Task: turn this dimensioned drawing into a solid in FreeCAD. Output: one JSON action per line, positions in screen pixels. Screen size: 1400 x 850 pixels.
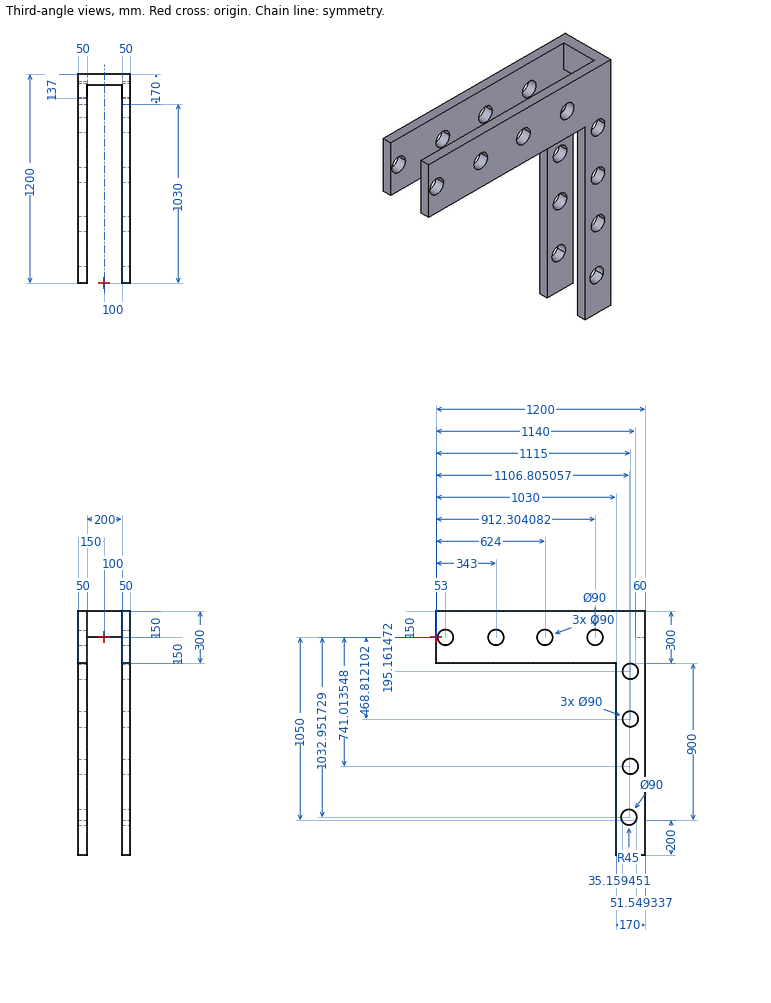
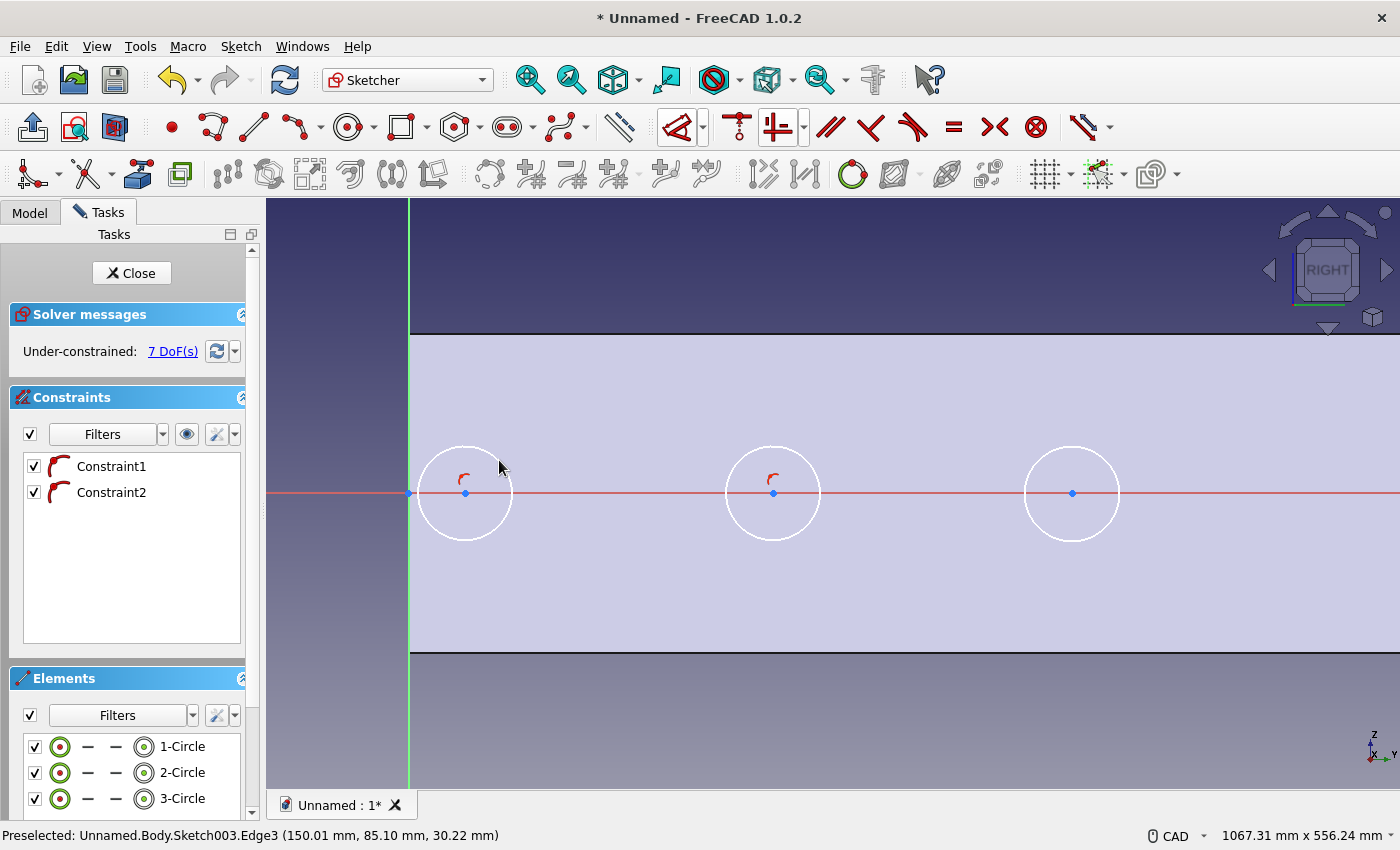
{"action": "left_click", "coordinate": [1105, 460]}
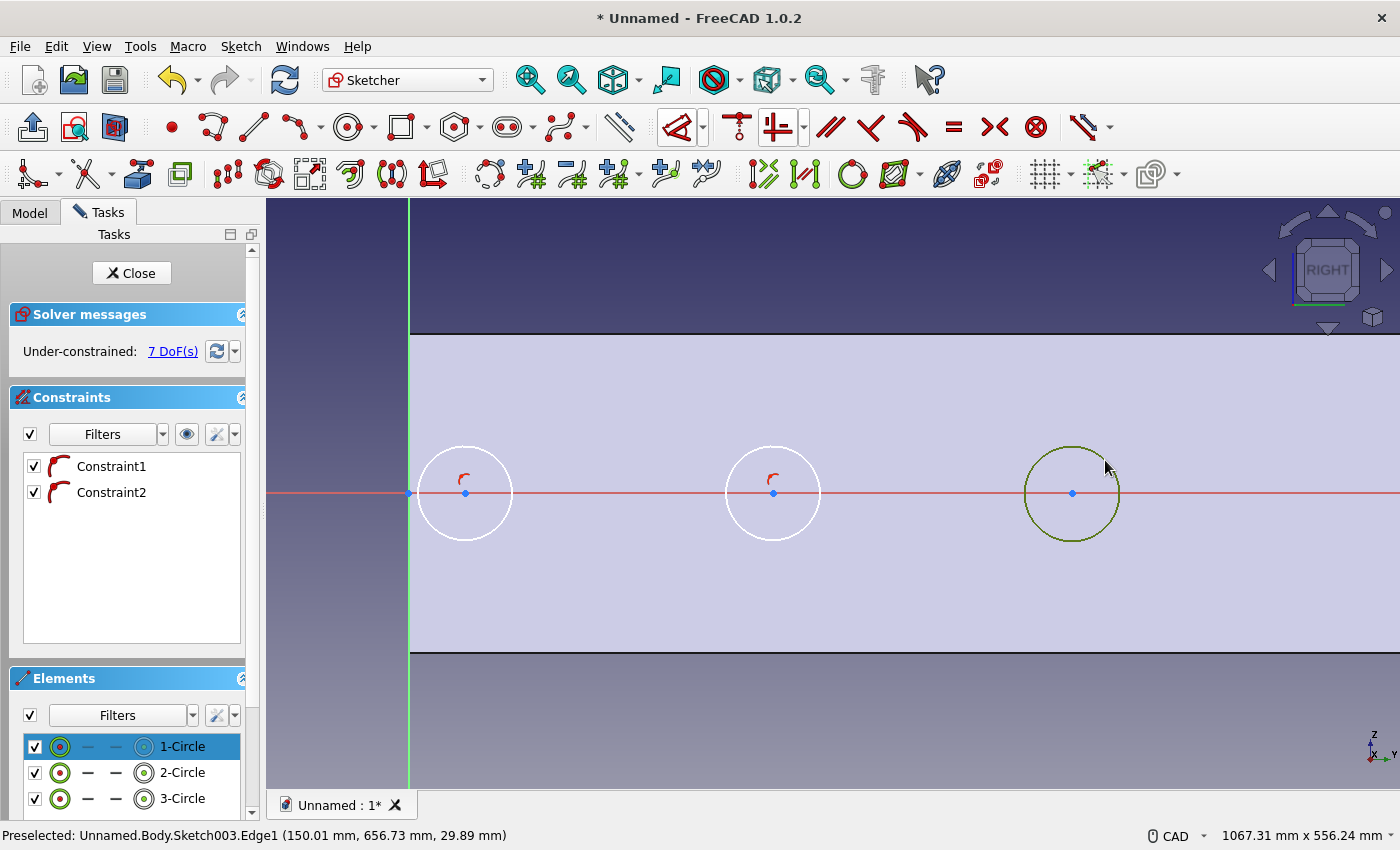
{"action": "left_click", "coordinate": [806, 460]}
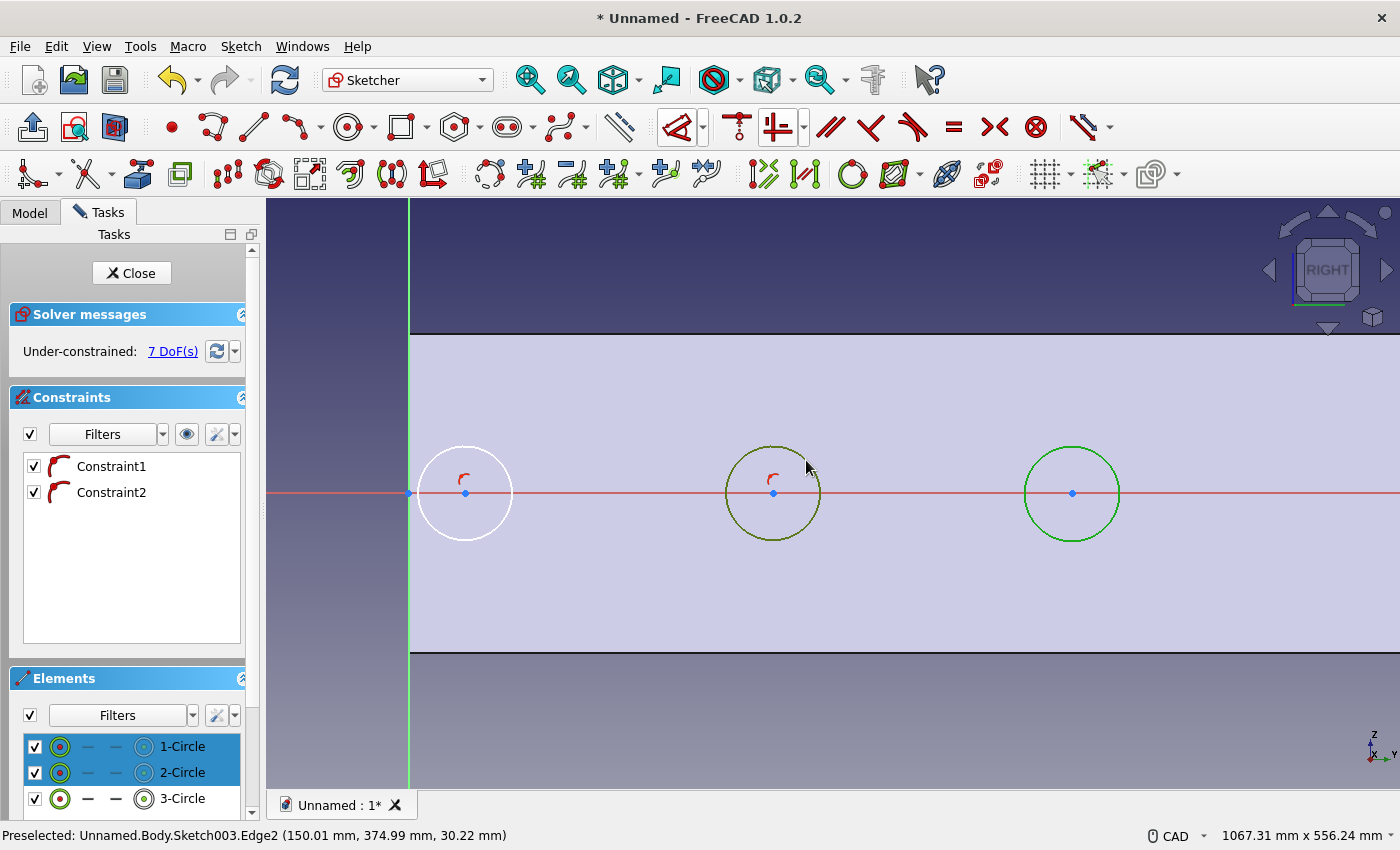
{"action": "left_click", "coordinate": [498, 460]}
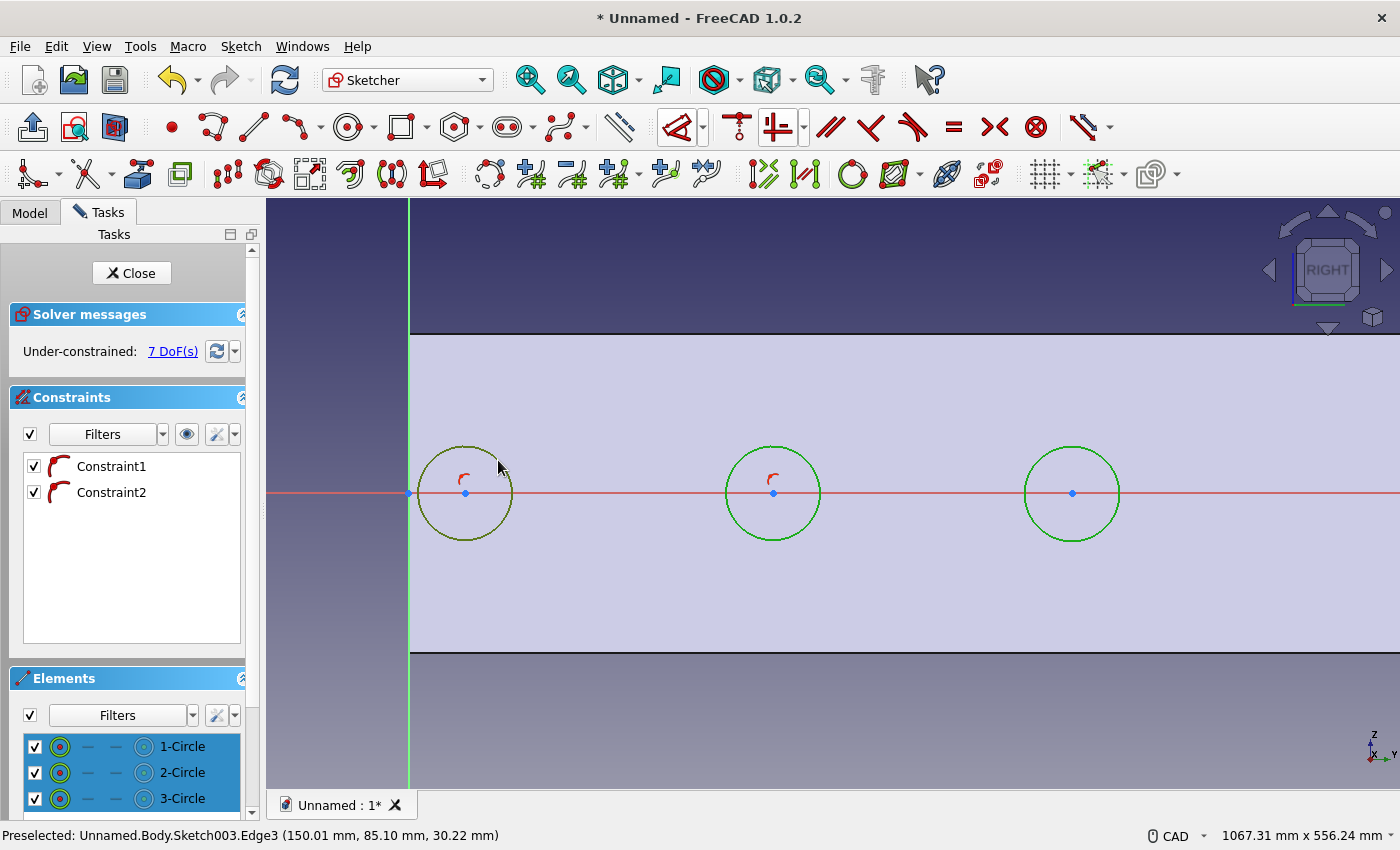
{"action": "left_click", "coordinate": [954, 128]}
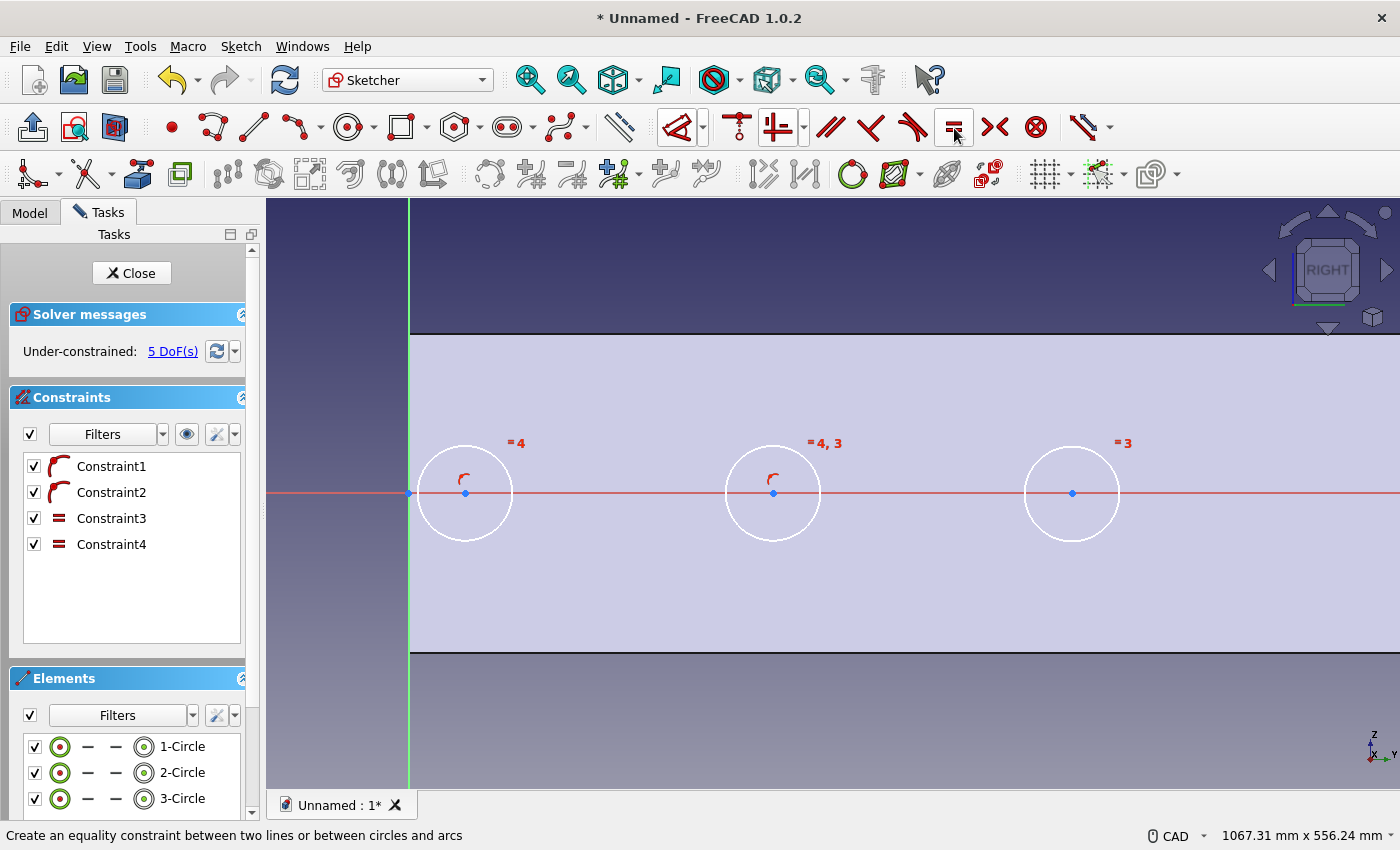
{"action": "left_click", "coordinate": [1072, 494]}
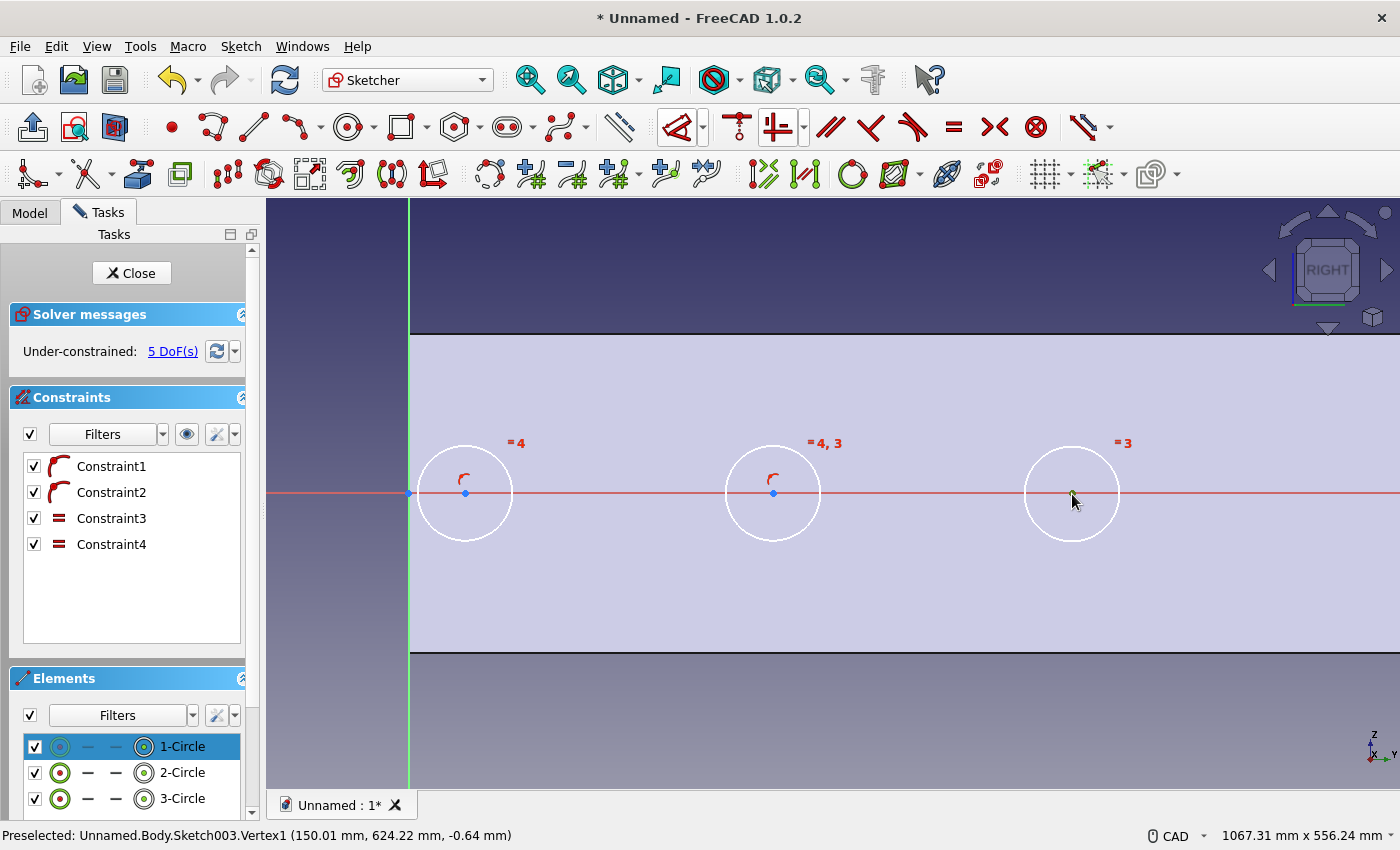
{"action": "left_click", "coordinate": [361, 493]}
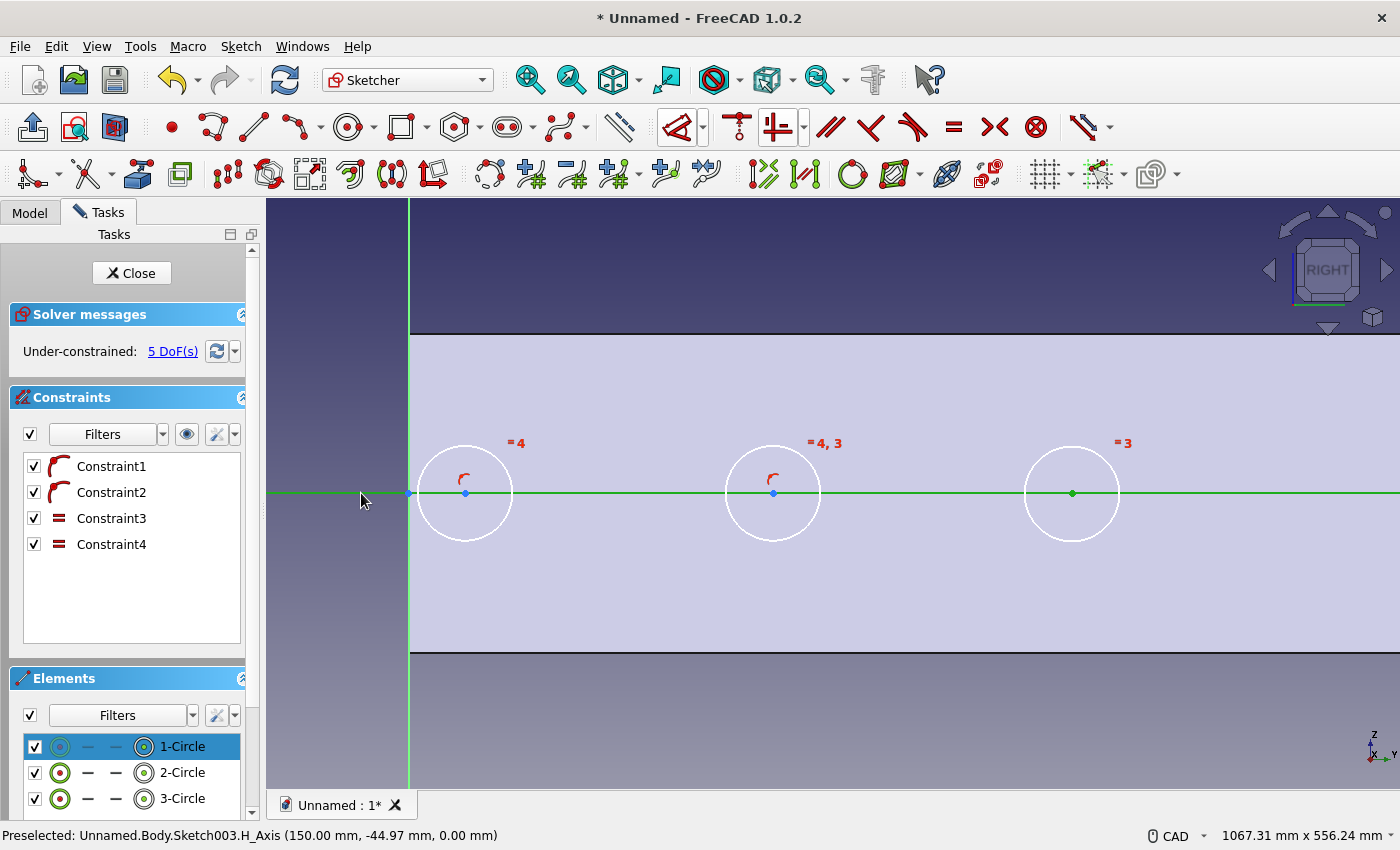
{"action": "left_click", "coordinate": [737, 128]}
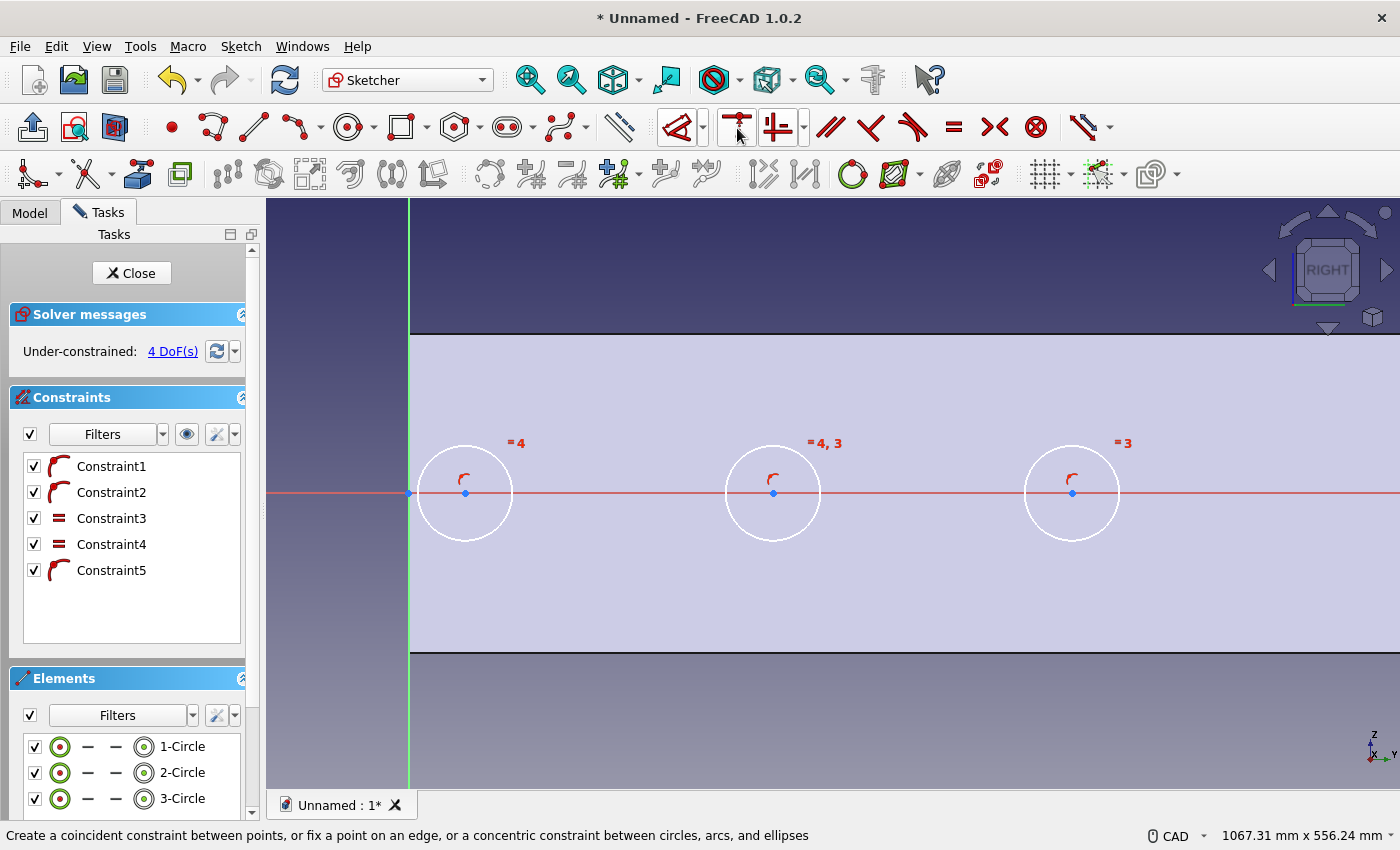
{"action": "left_click", "coordinate": [1105, 460]}